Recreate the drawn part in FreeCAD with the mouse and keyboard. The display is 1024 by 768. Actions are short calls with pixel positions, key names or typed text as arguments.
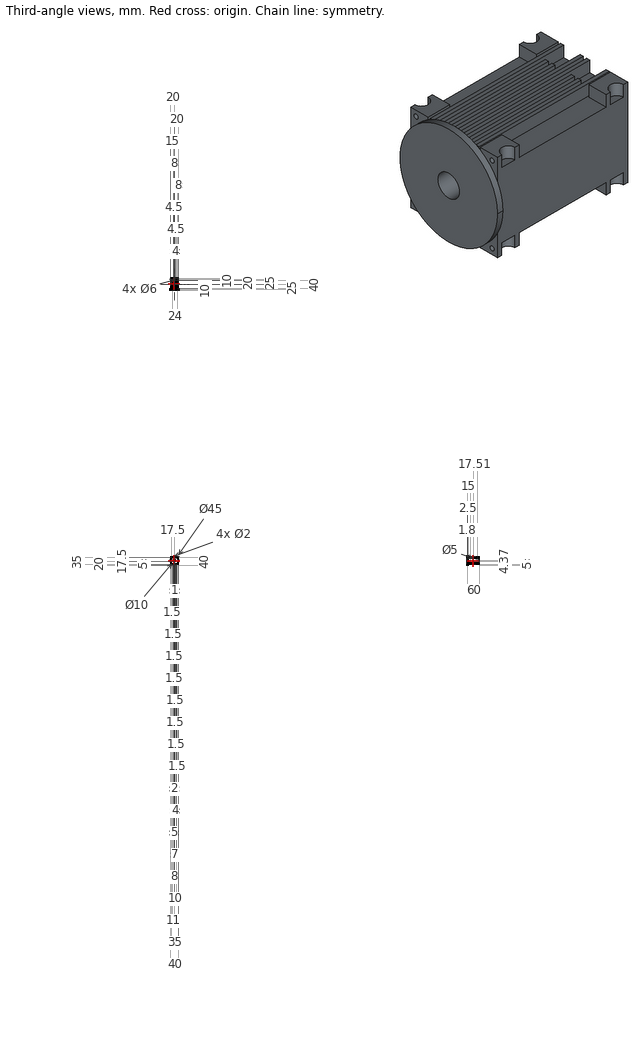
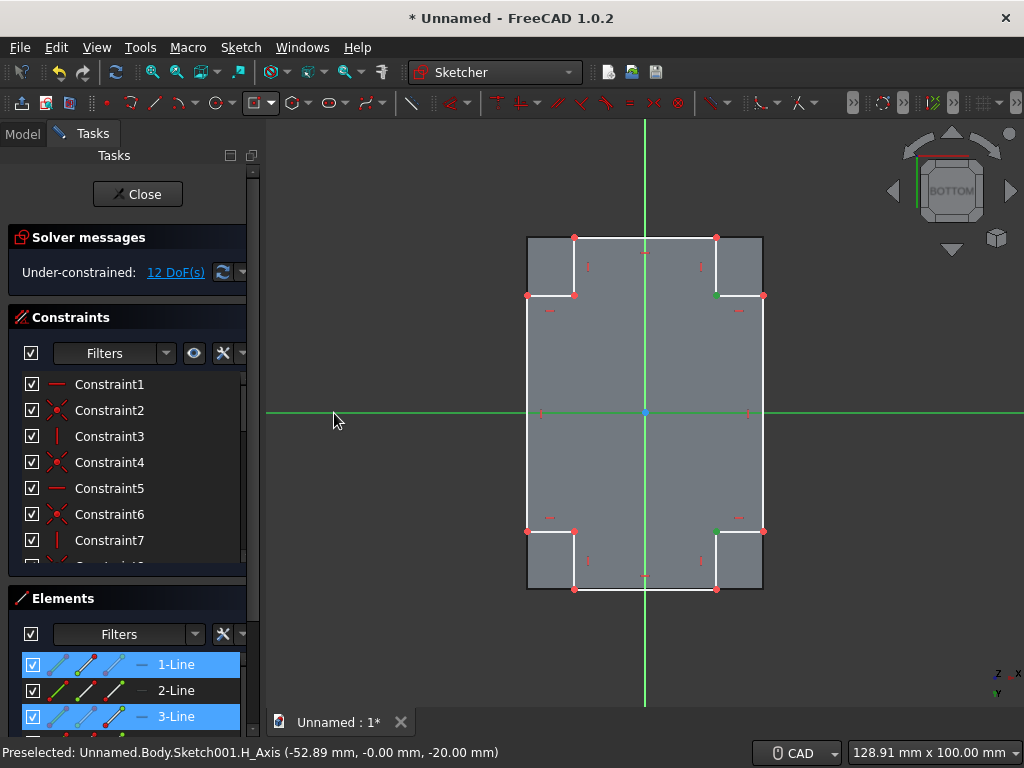
click(654, 104)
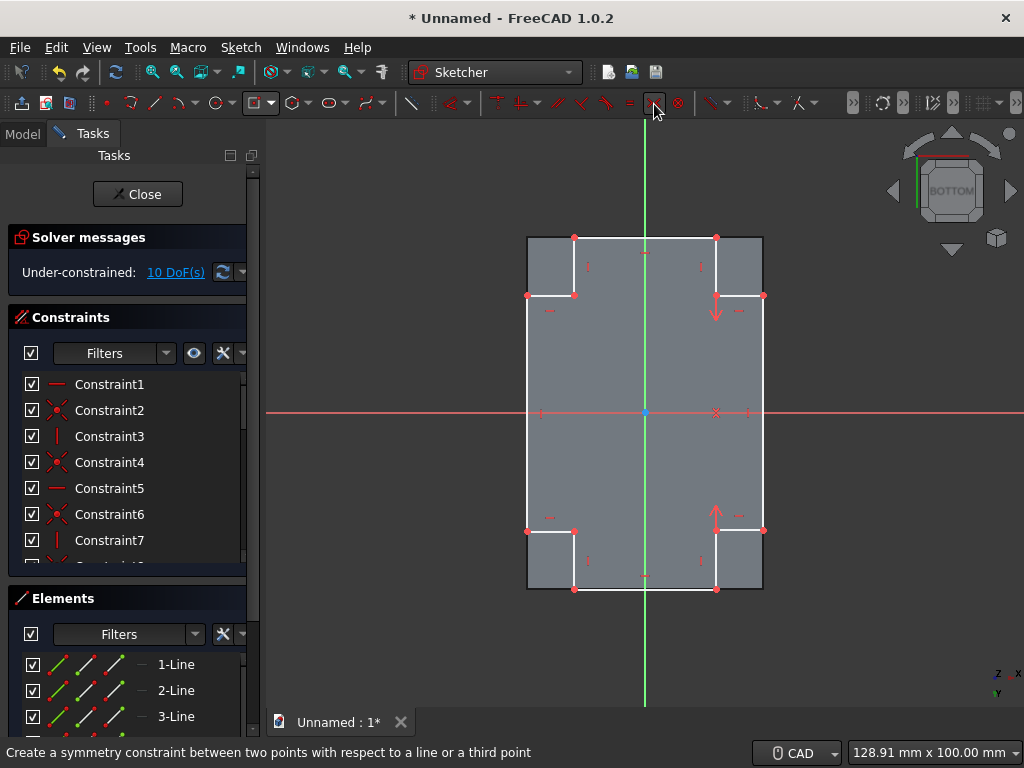
click(716, 296)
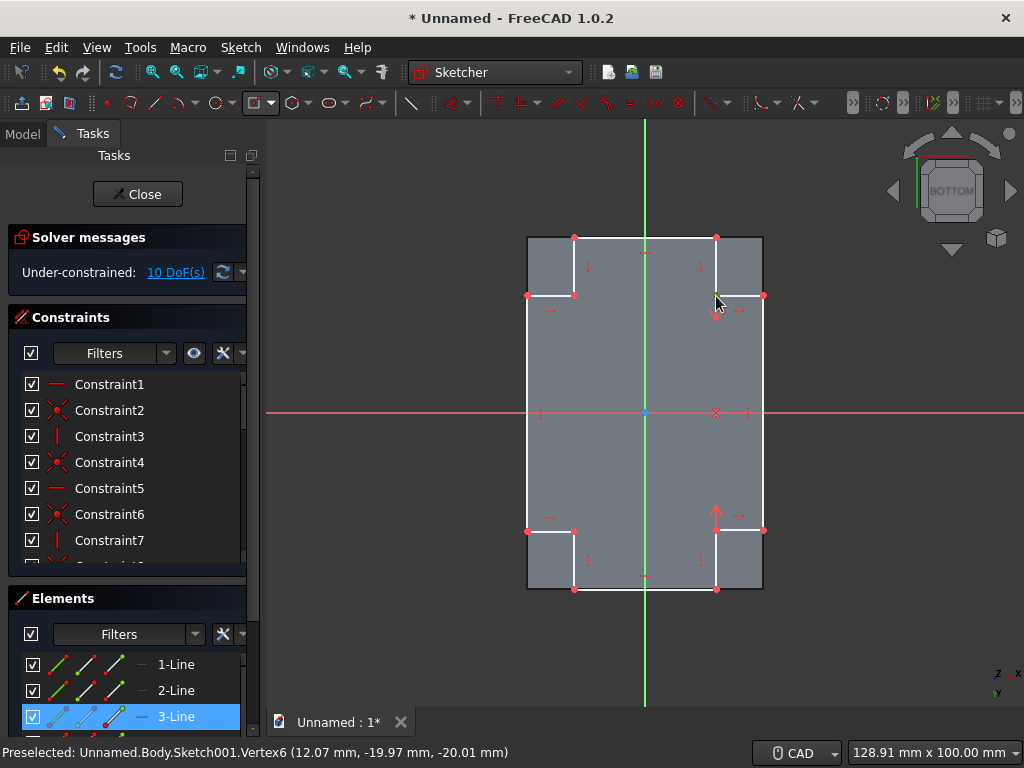
click(574, 296)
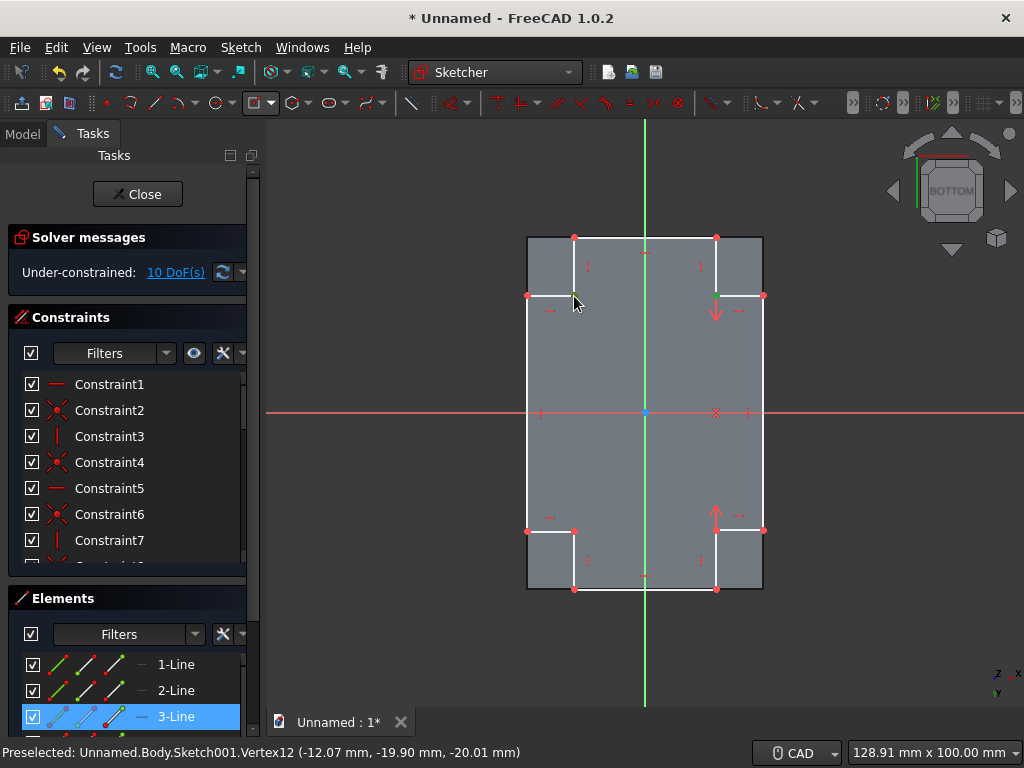
click(645, 641)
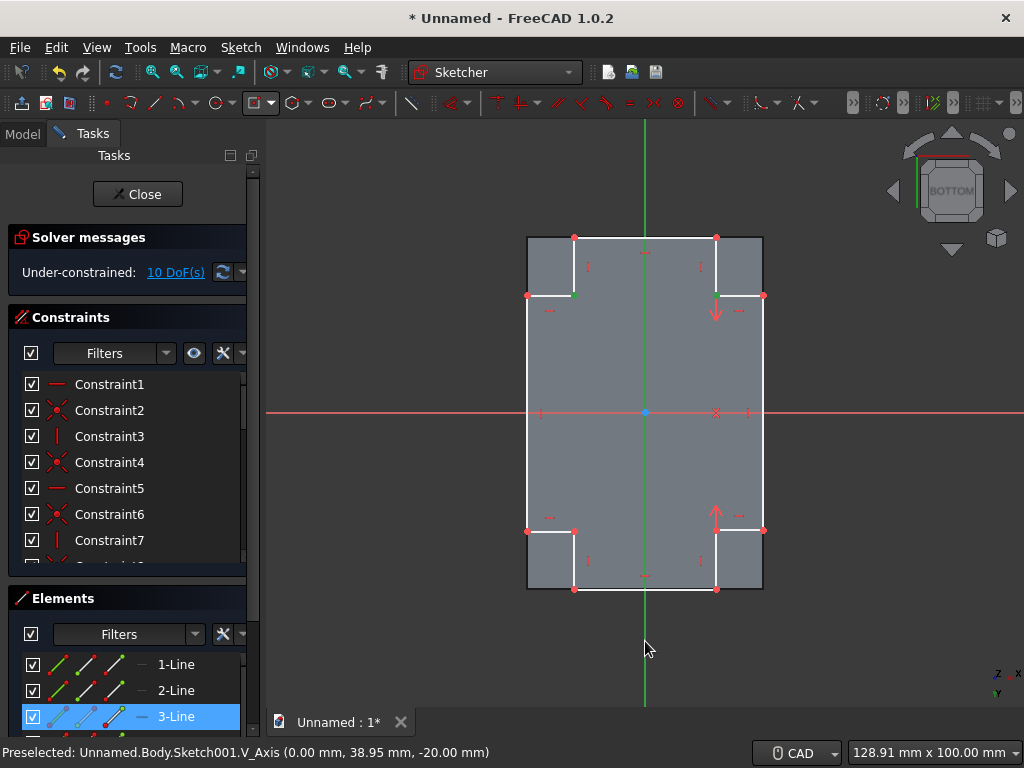
click(654, 104)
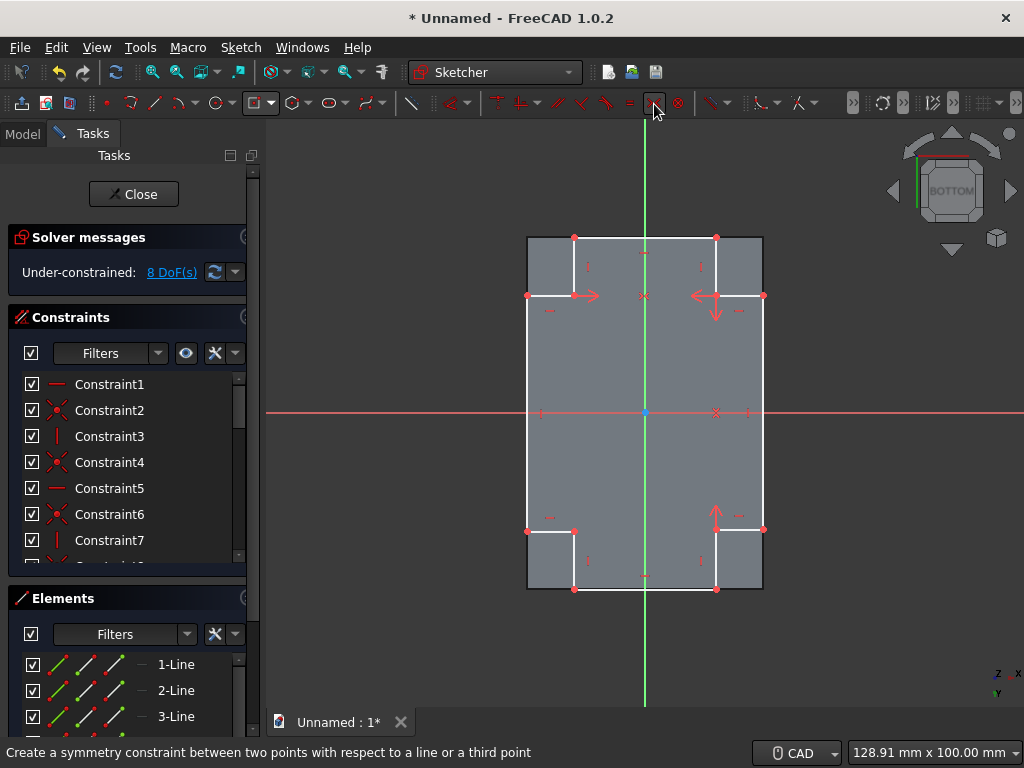
click(763, 530)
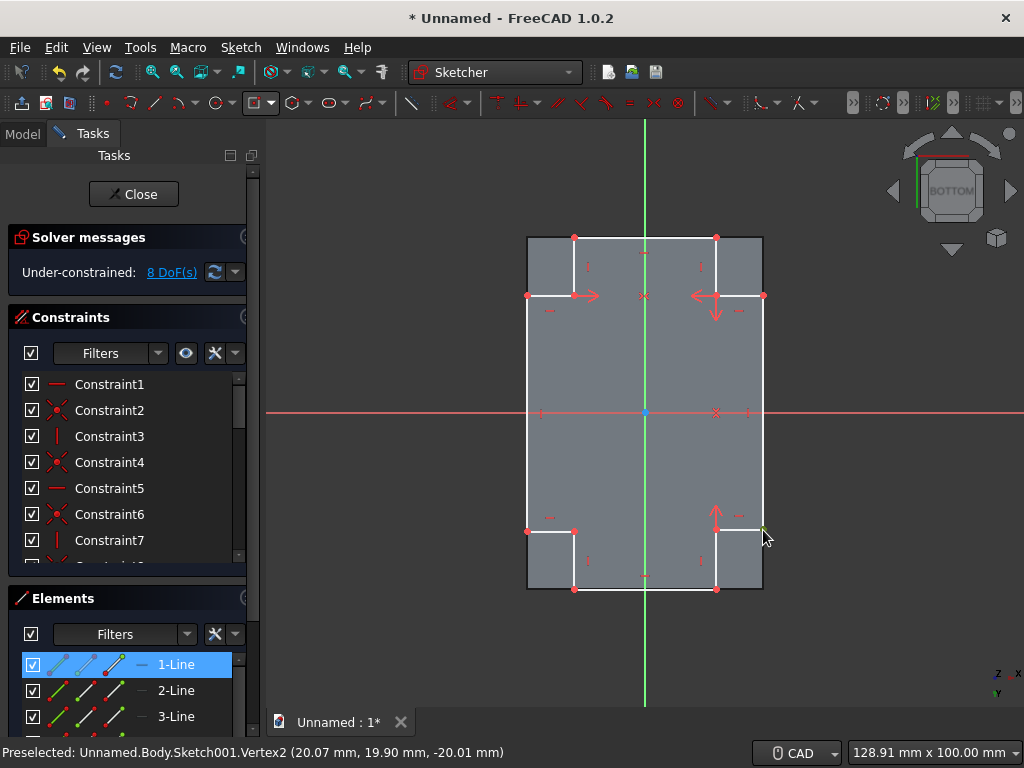
click(527, 532)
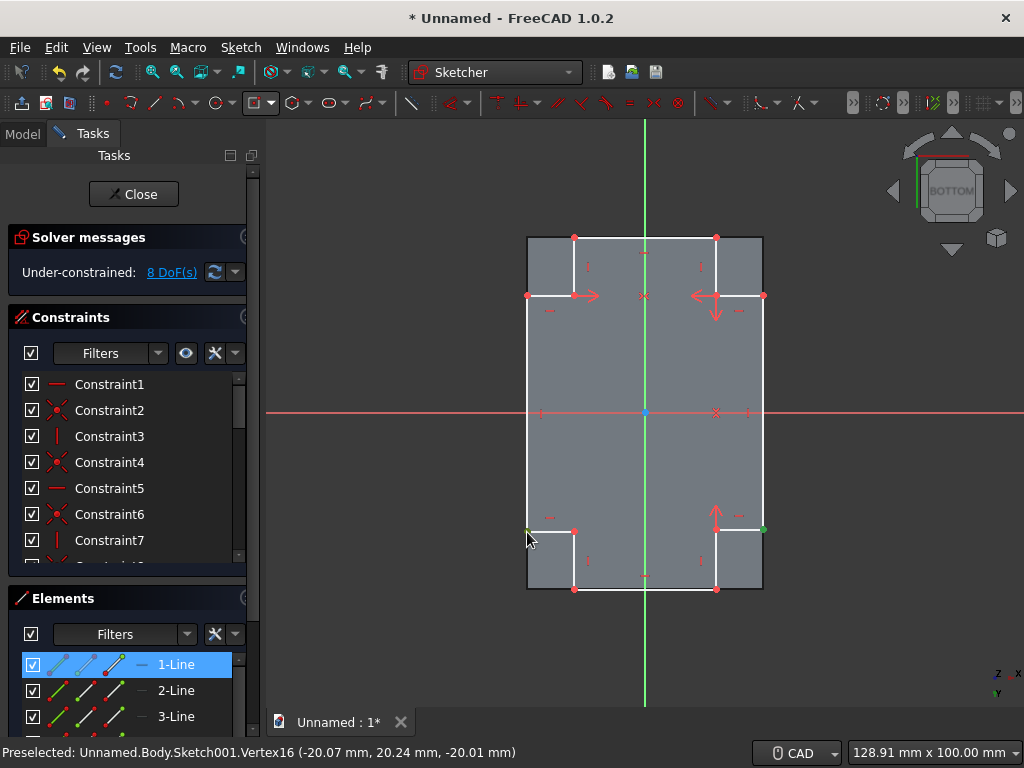
click(645, 641)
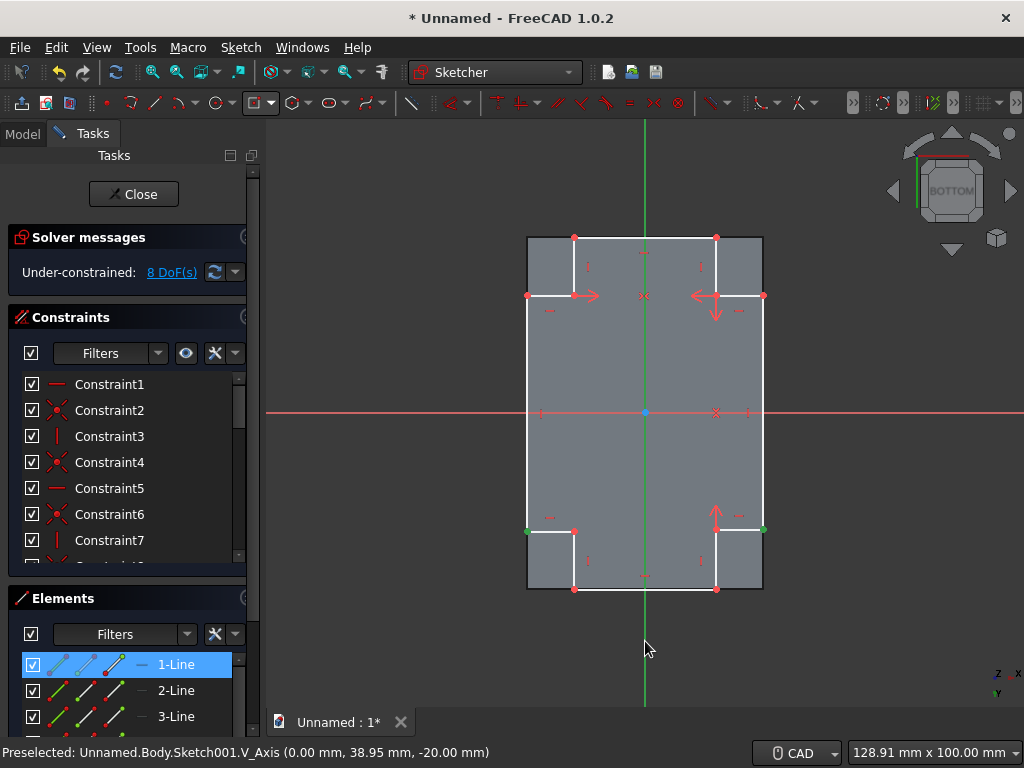
click(654, 104)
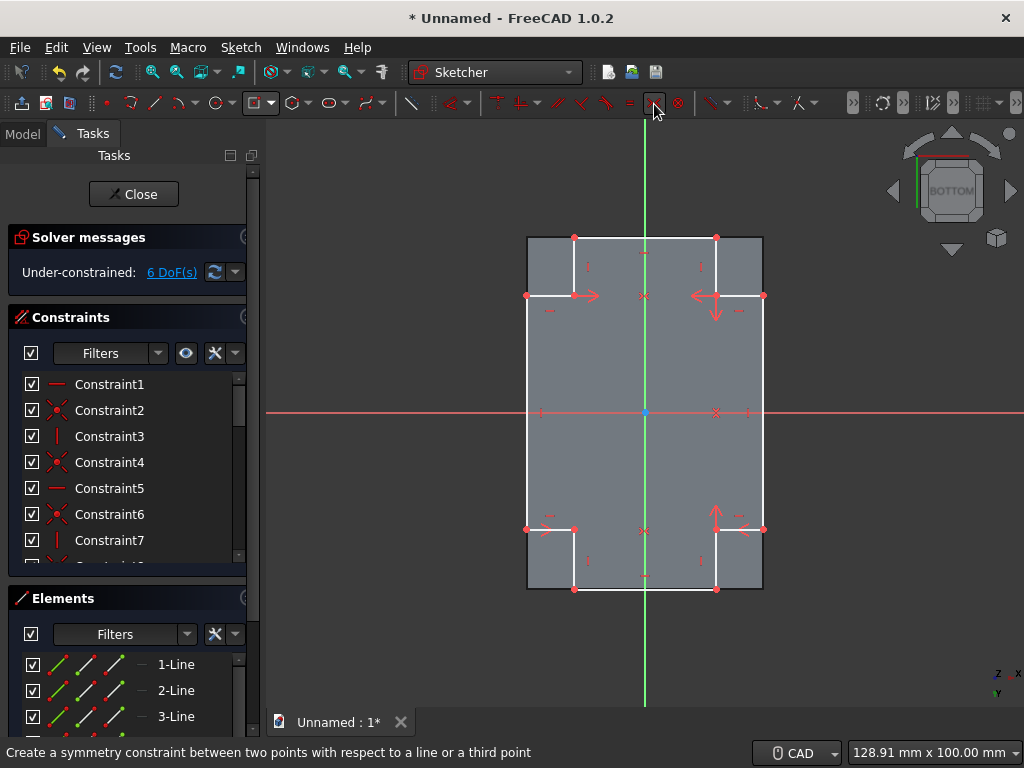
click(574, 238)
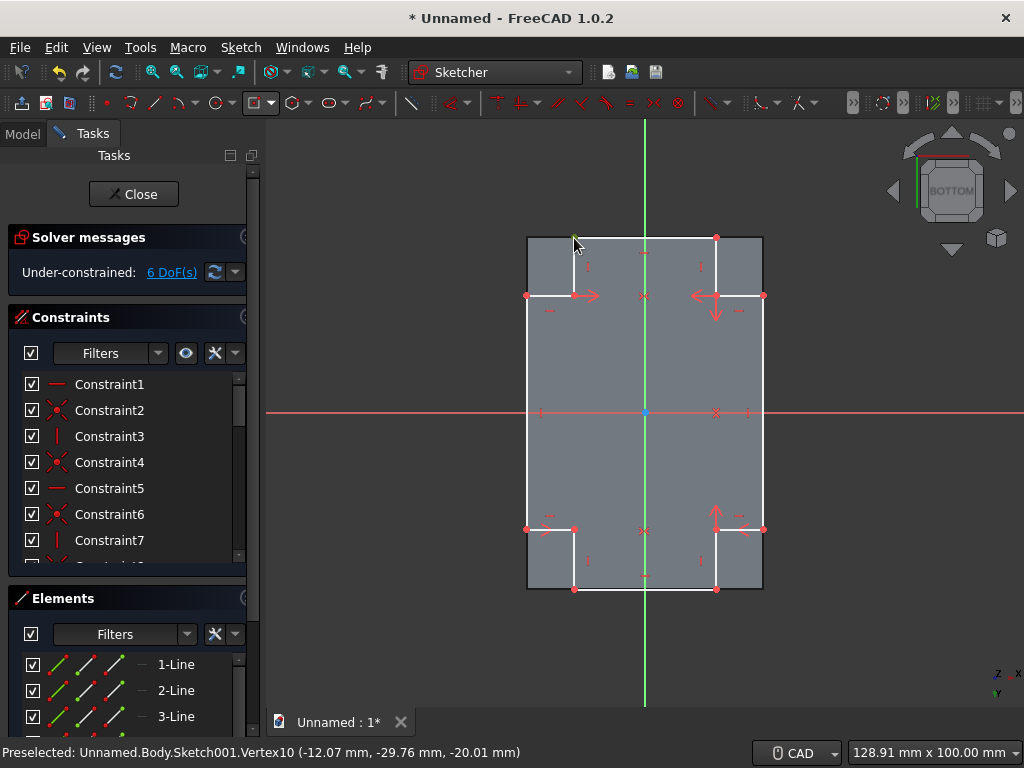
click(574, 590)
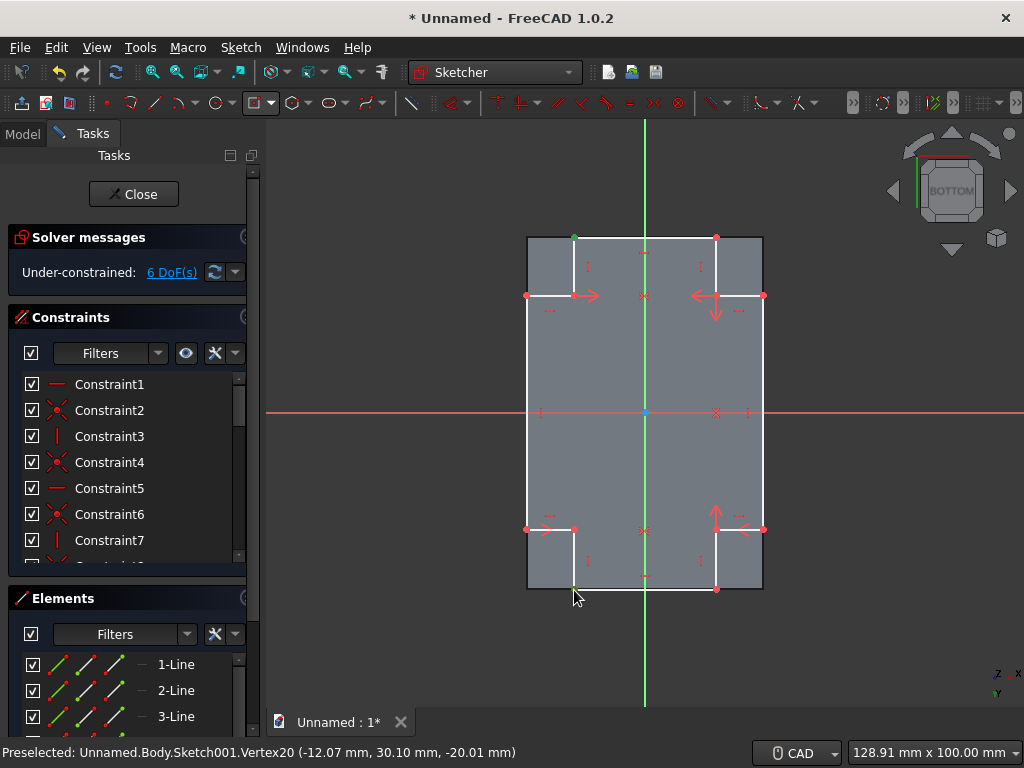
click(334, 413)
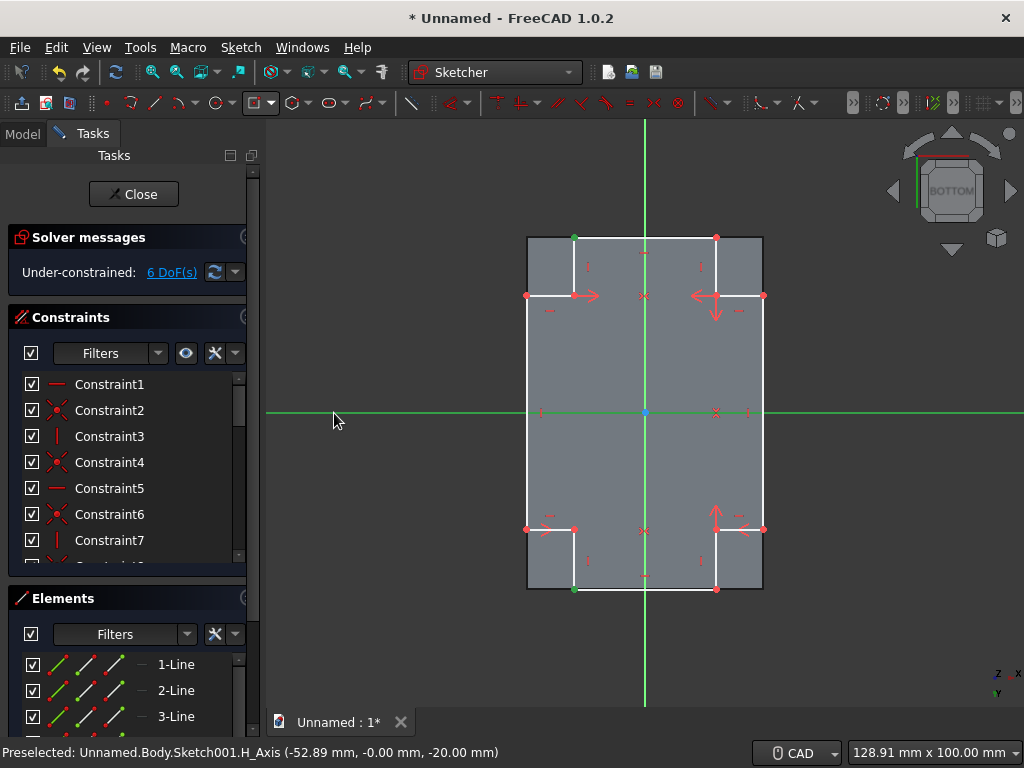
click(654, 104)